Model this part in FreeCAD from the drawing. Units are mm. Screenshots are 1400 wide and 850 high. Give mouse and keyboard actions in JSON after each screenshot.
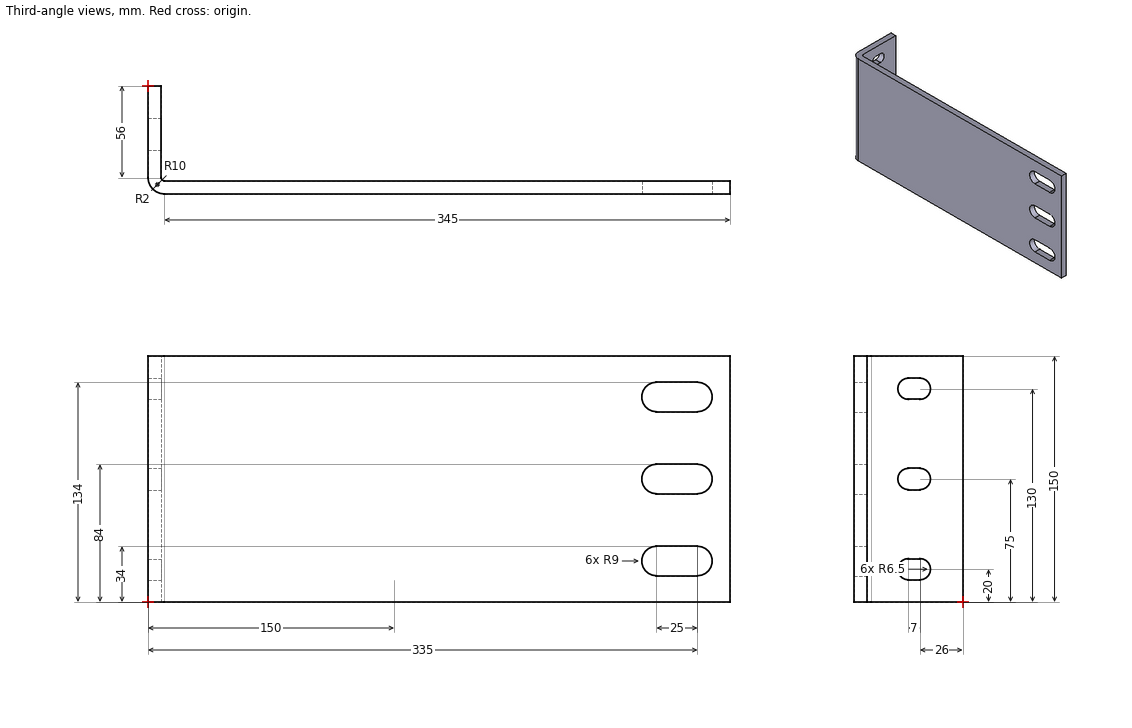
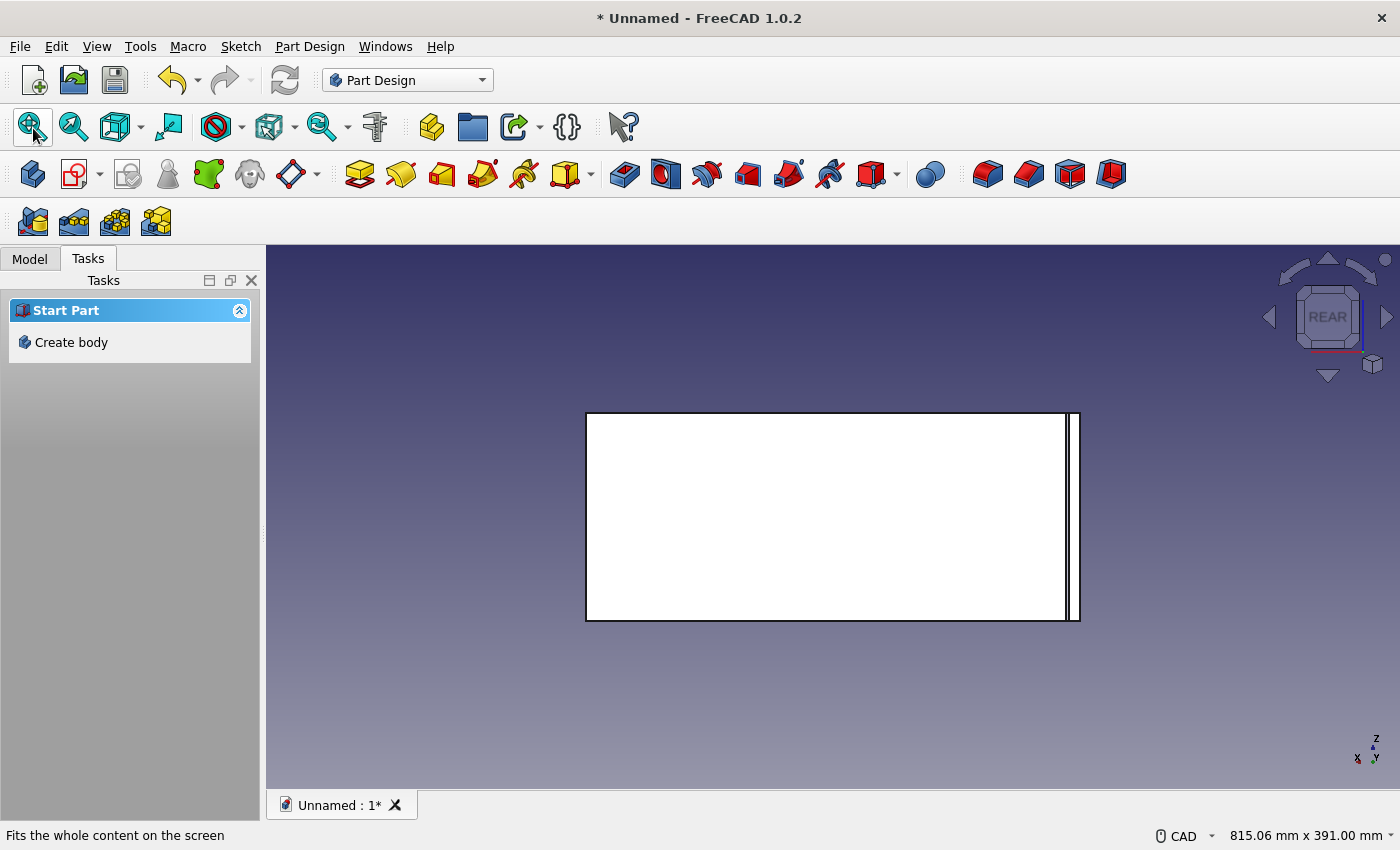
{"action": "left_click", "coordinate": [33, 128]}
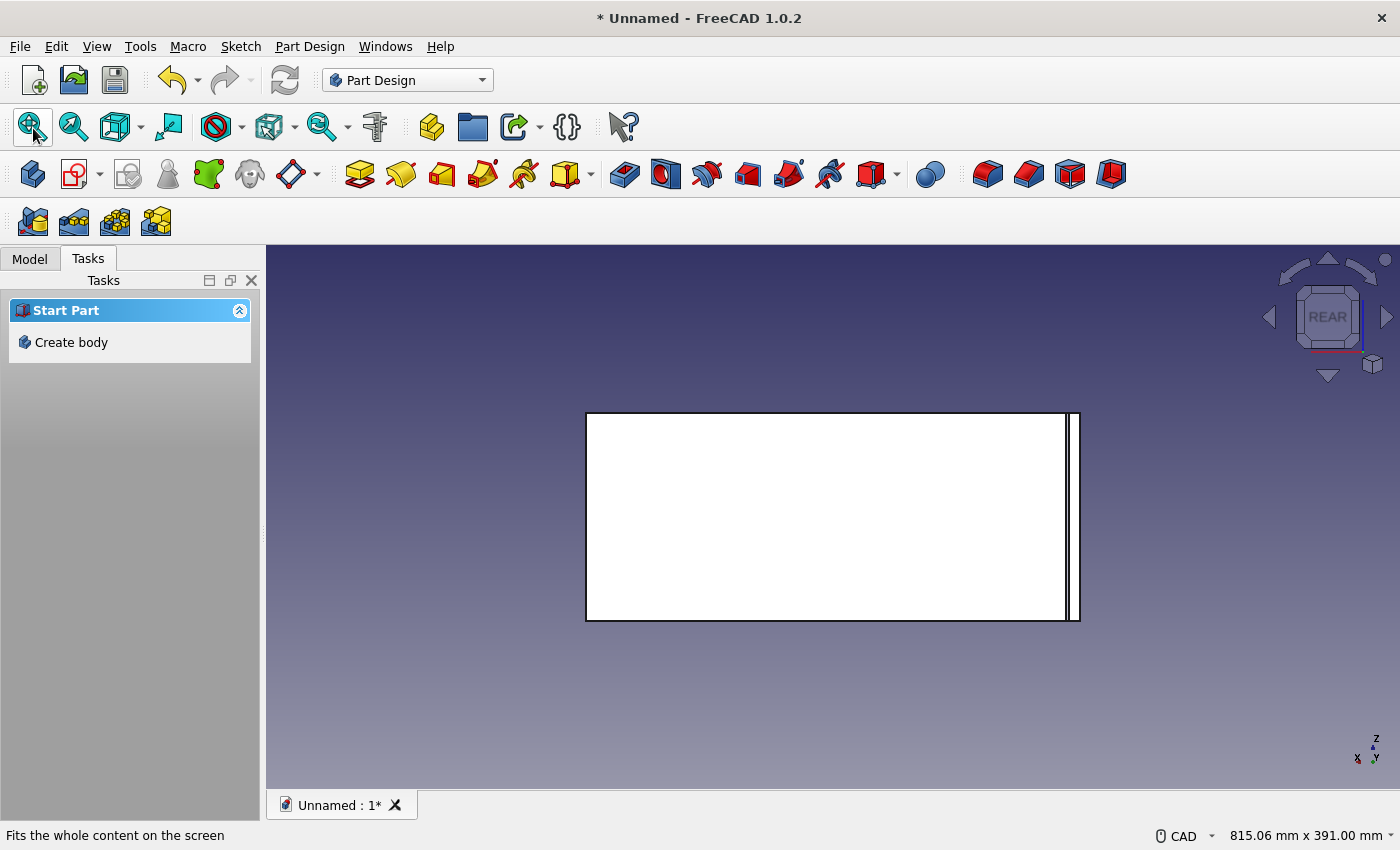
{"action": "left_click", "coordinate": [757, 516]}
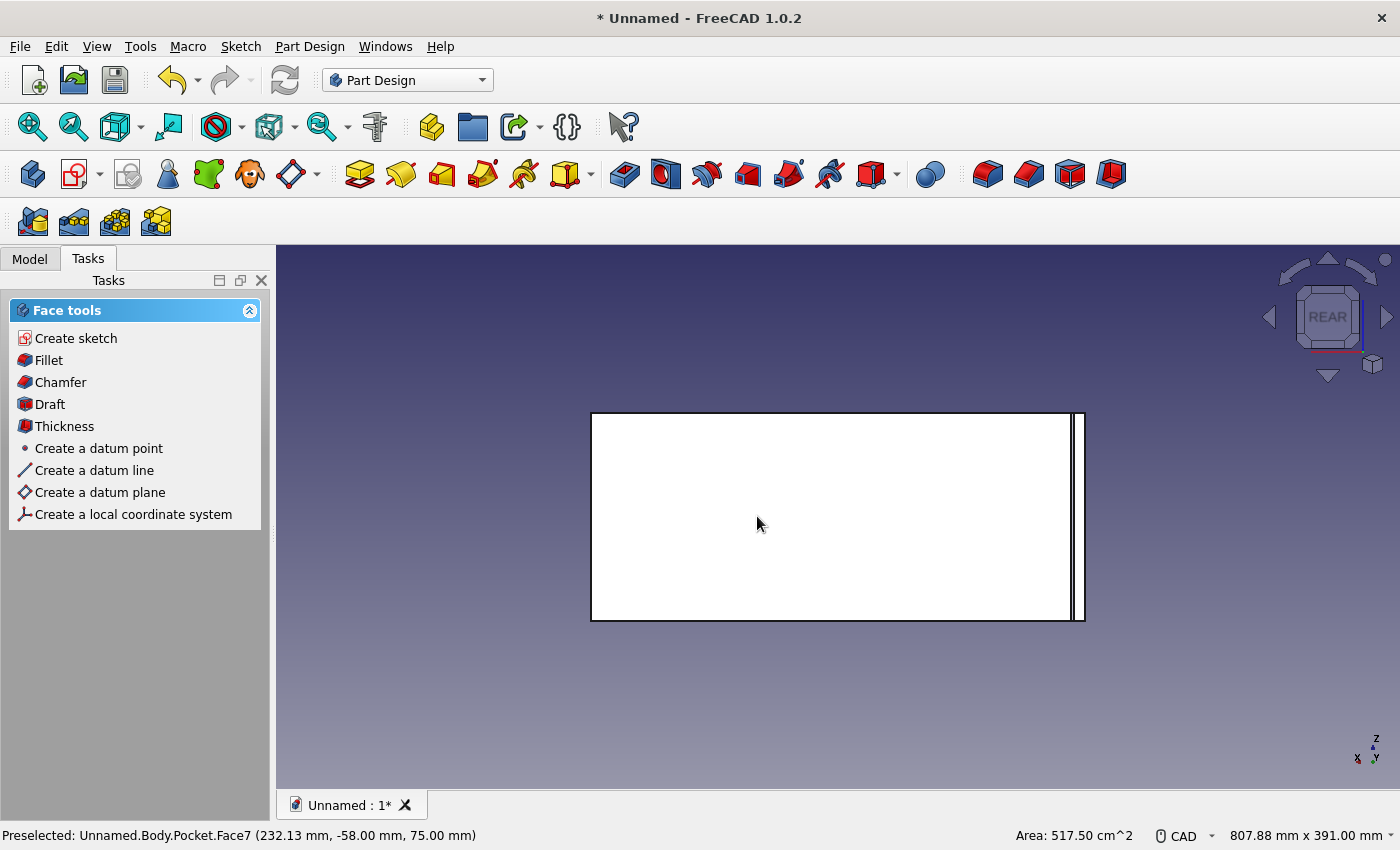
{"action": "left_click", "coordinate": [74, 174]}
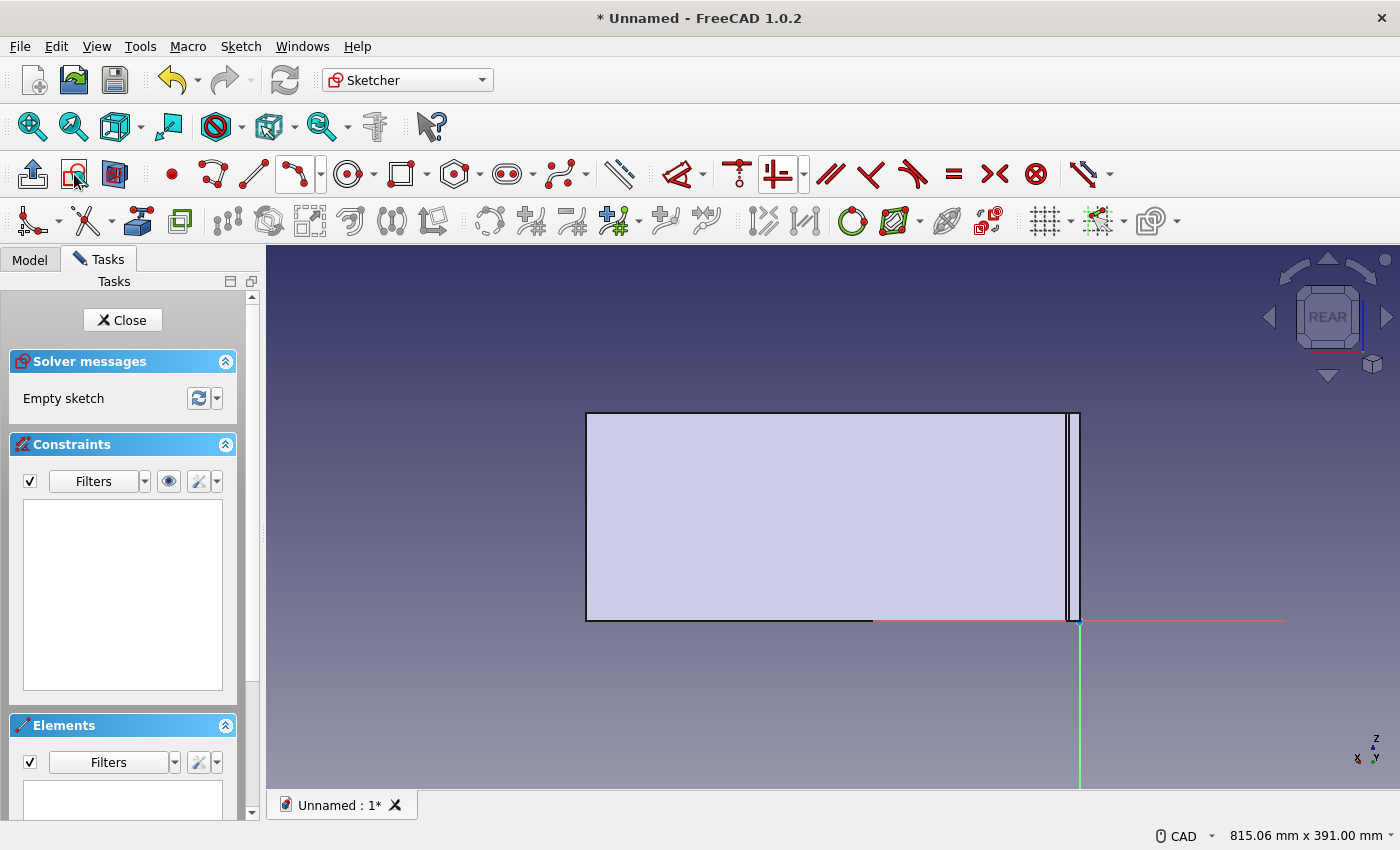
{"action": "left_click", "coordinate": [115, 174]}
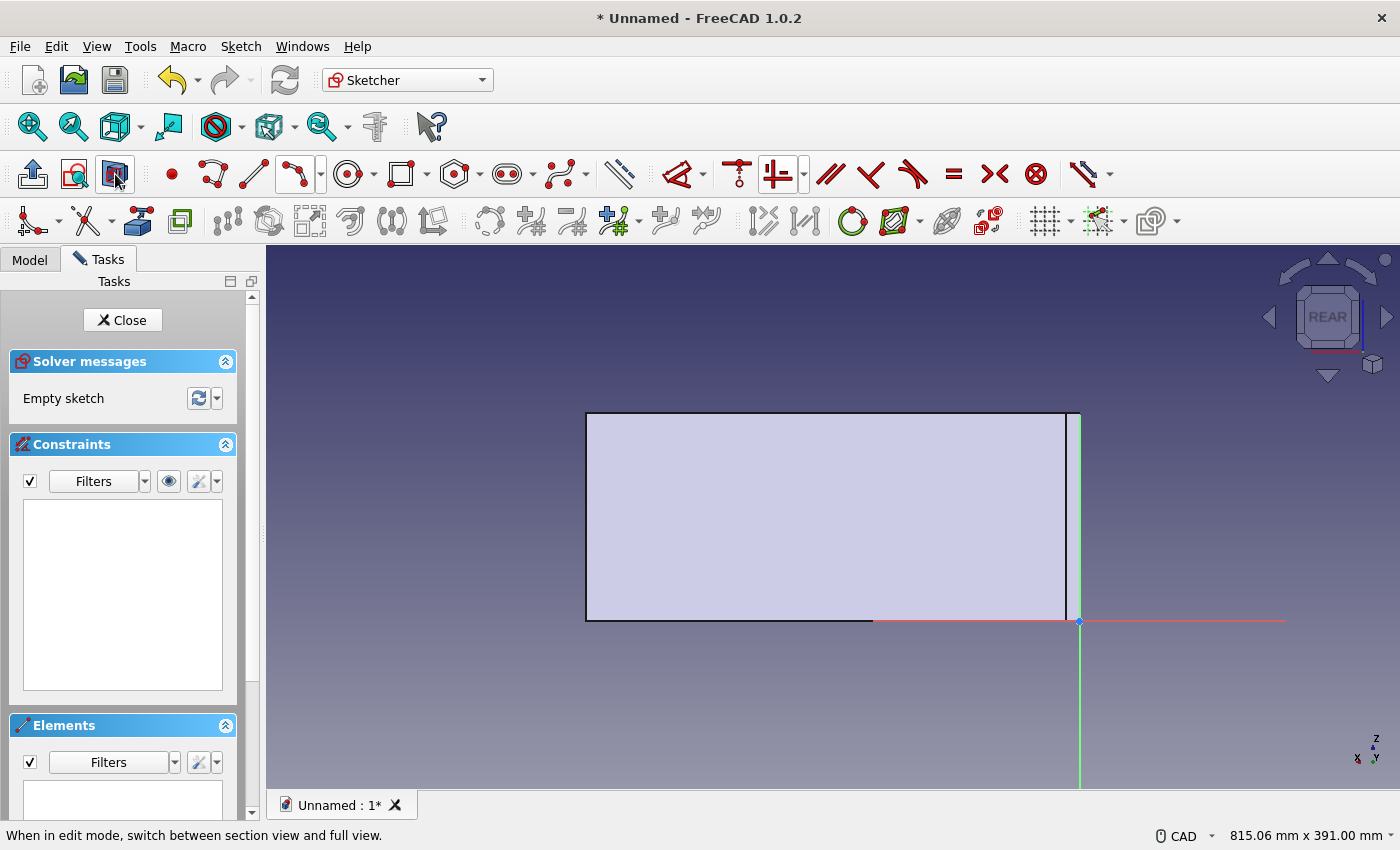
{"action": "scroll", "coordinate": [523, 517], "scroll_direction": "up", "scroll_amount": 4}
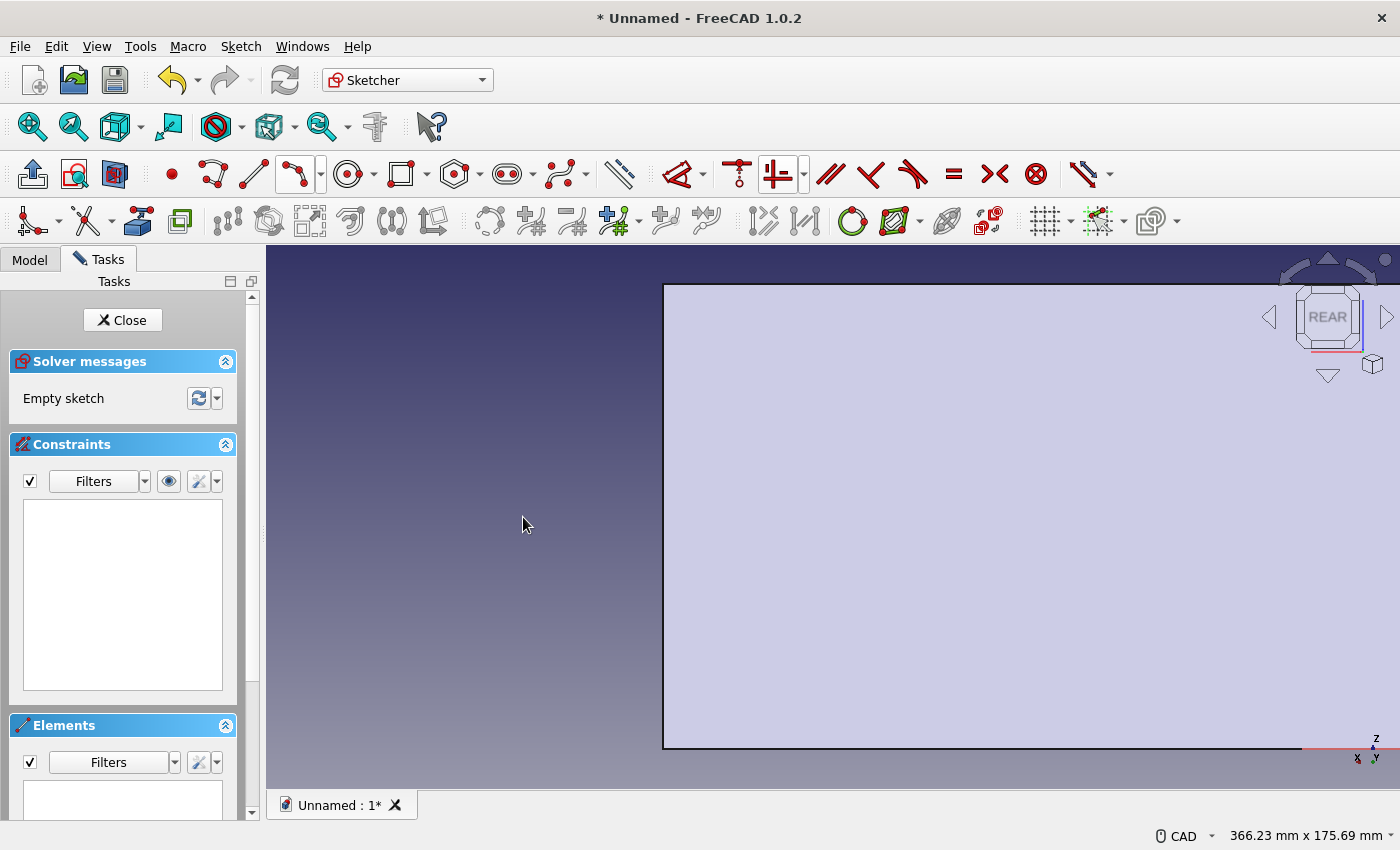
{"action": "left_click", "coordinate": [506, 174]}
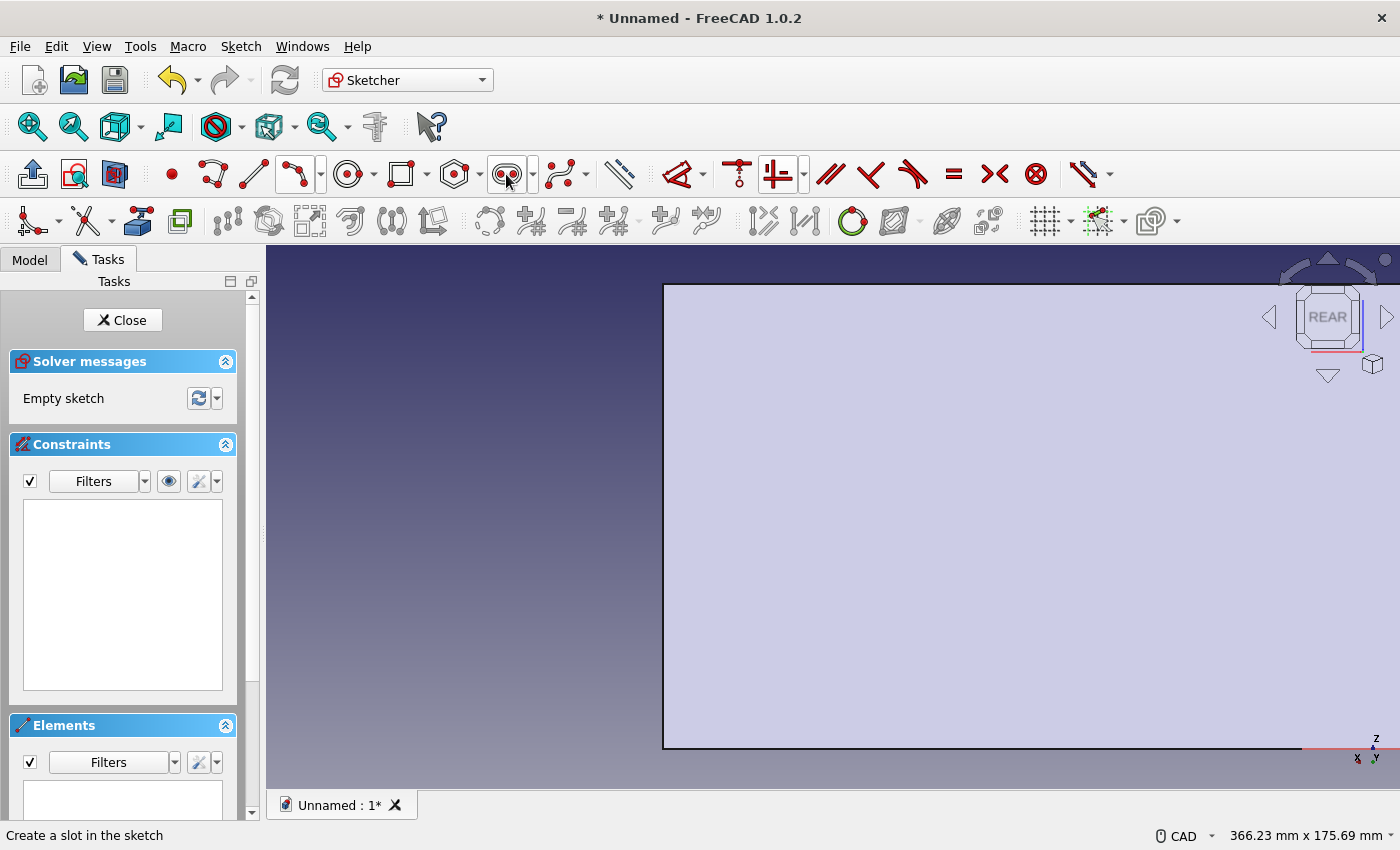
{"action": "left_click", "coordinate": [725, 671]}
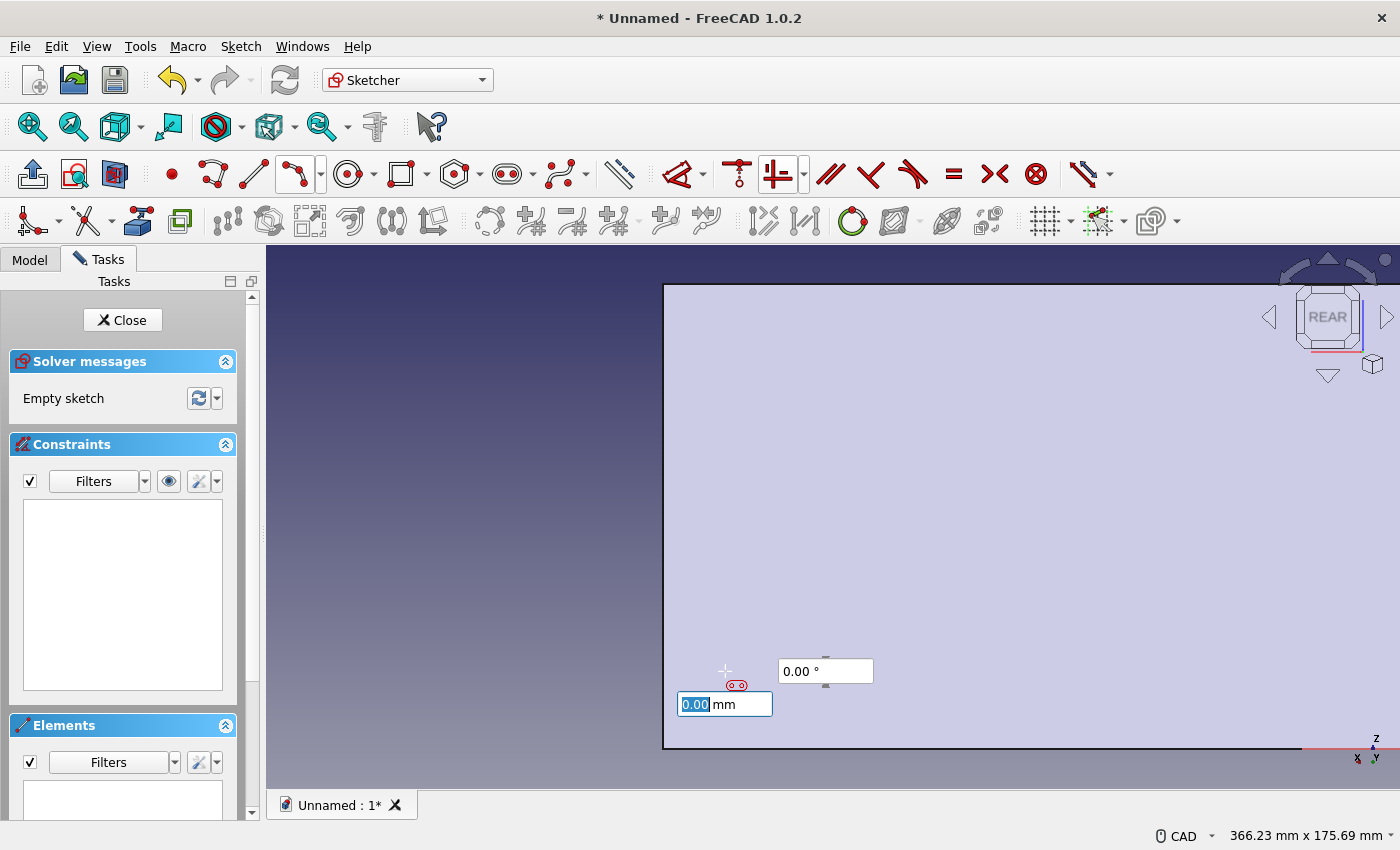
{"action": "left_click", "coordinate": [802, 671]}